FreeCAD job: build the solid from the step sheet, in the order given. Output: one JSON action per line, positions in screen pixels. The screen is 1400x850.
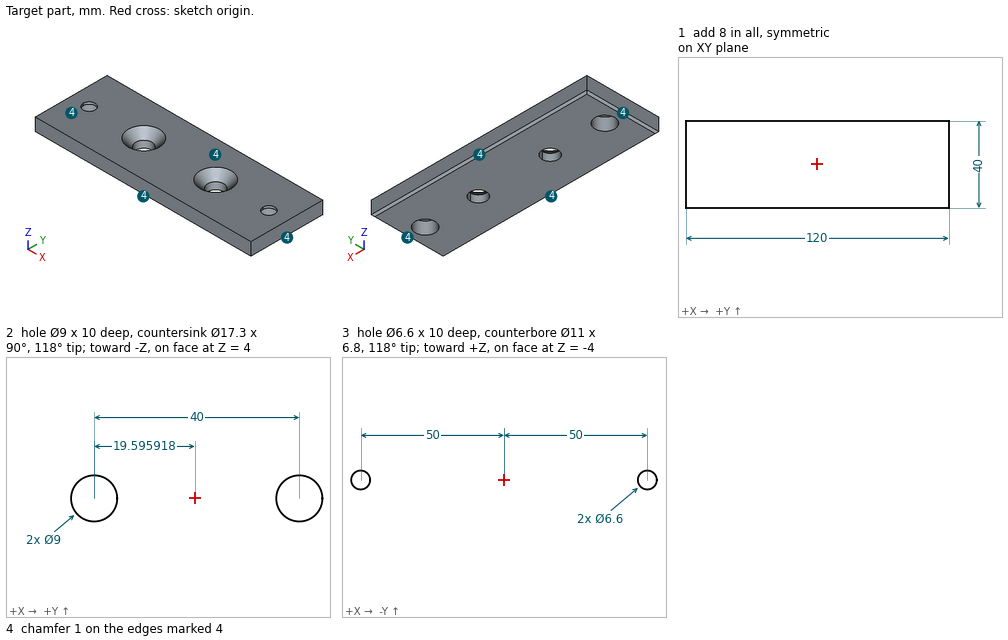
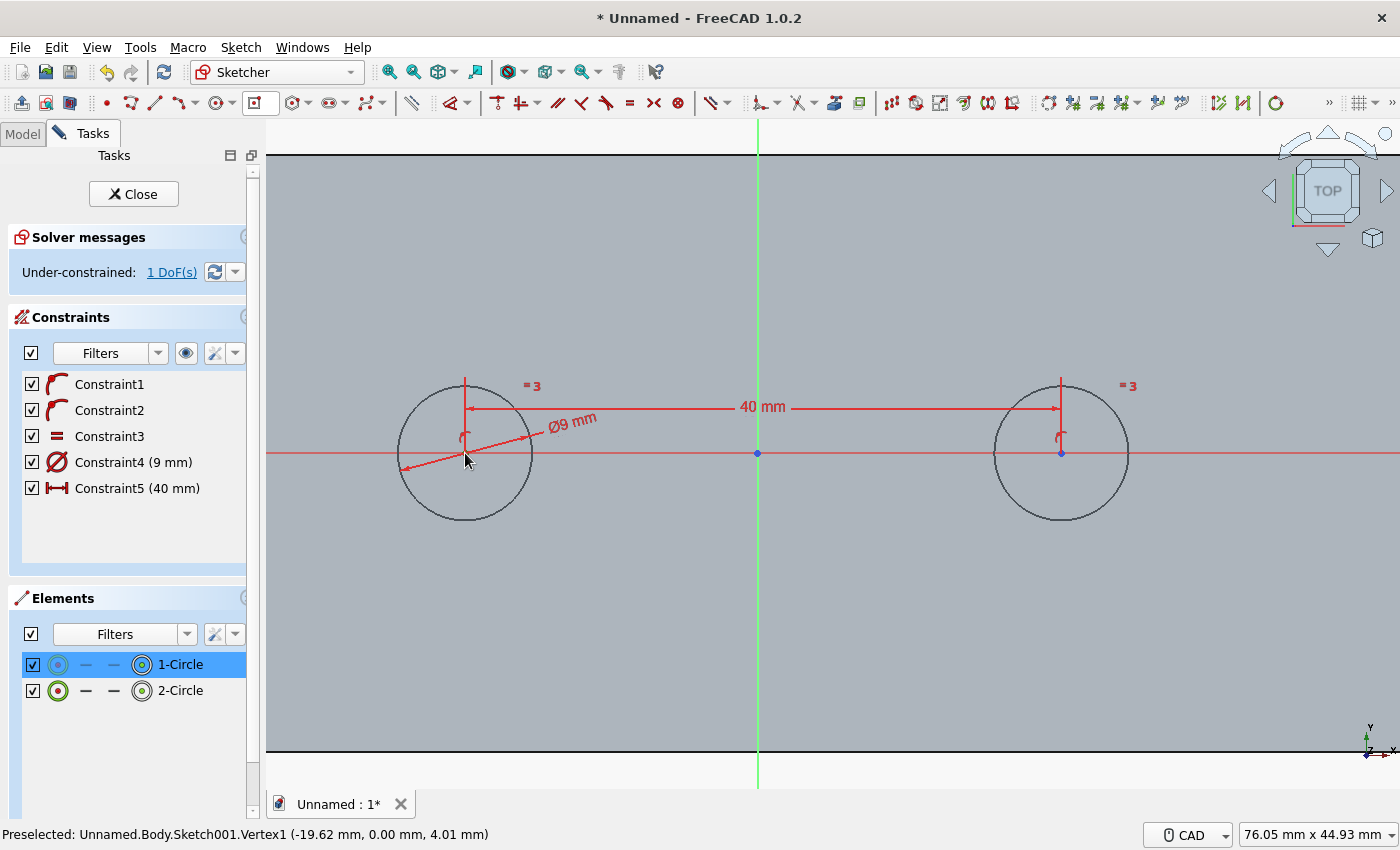
{"action": "key", "text": "l"}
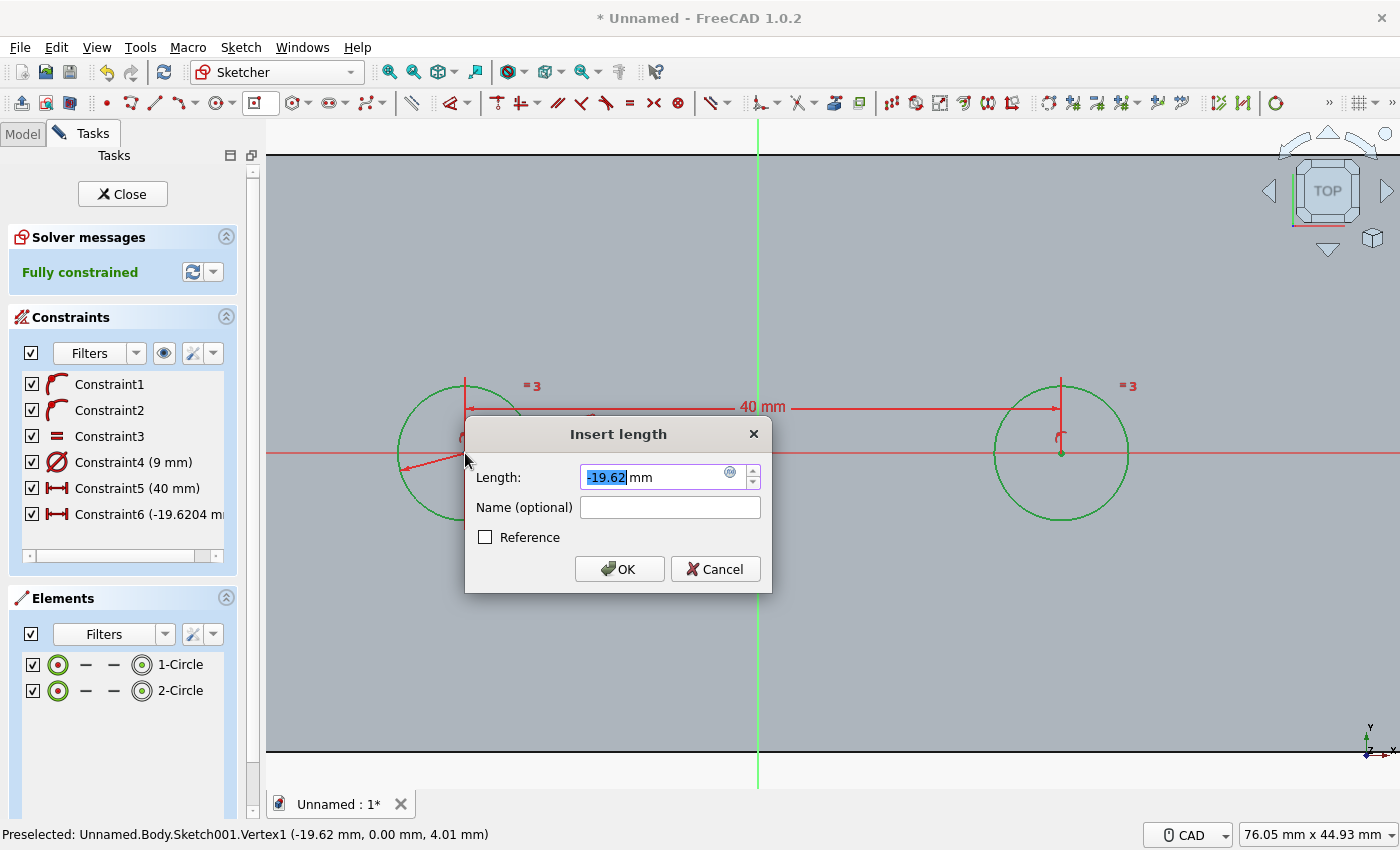
{"action": "type", "text": "-19.595918"}
{"action": "key", "text": "Return"}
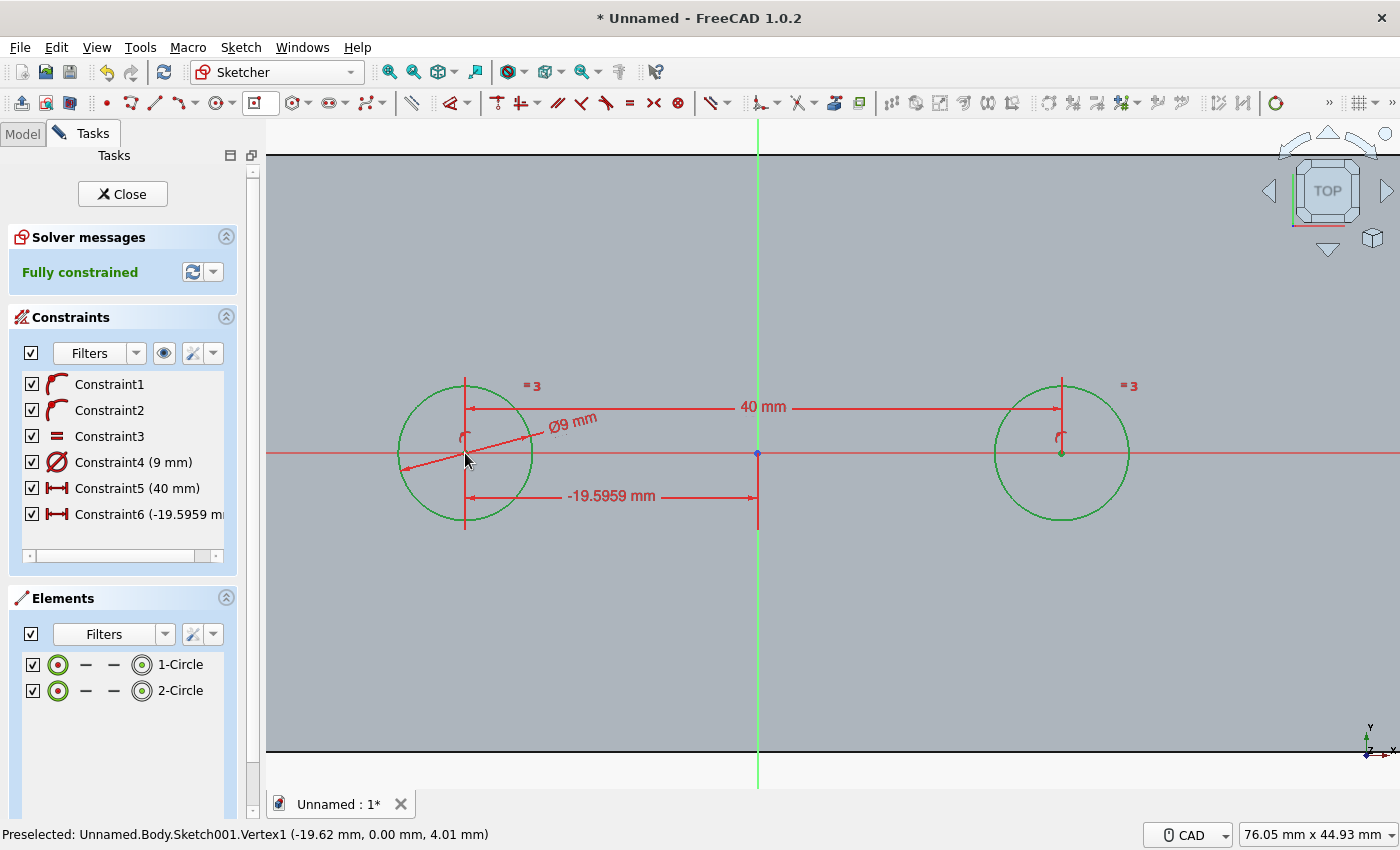
{"action": "left_click", "coordinate": [123, 194]}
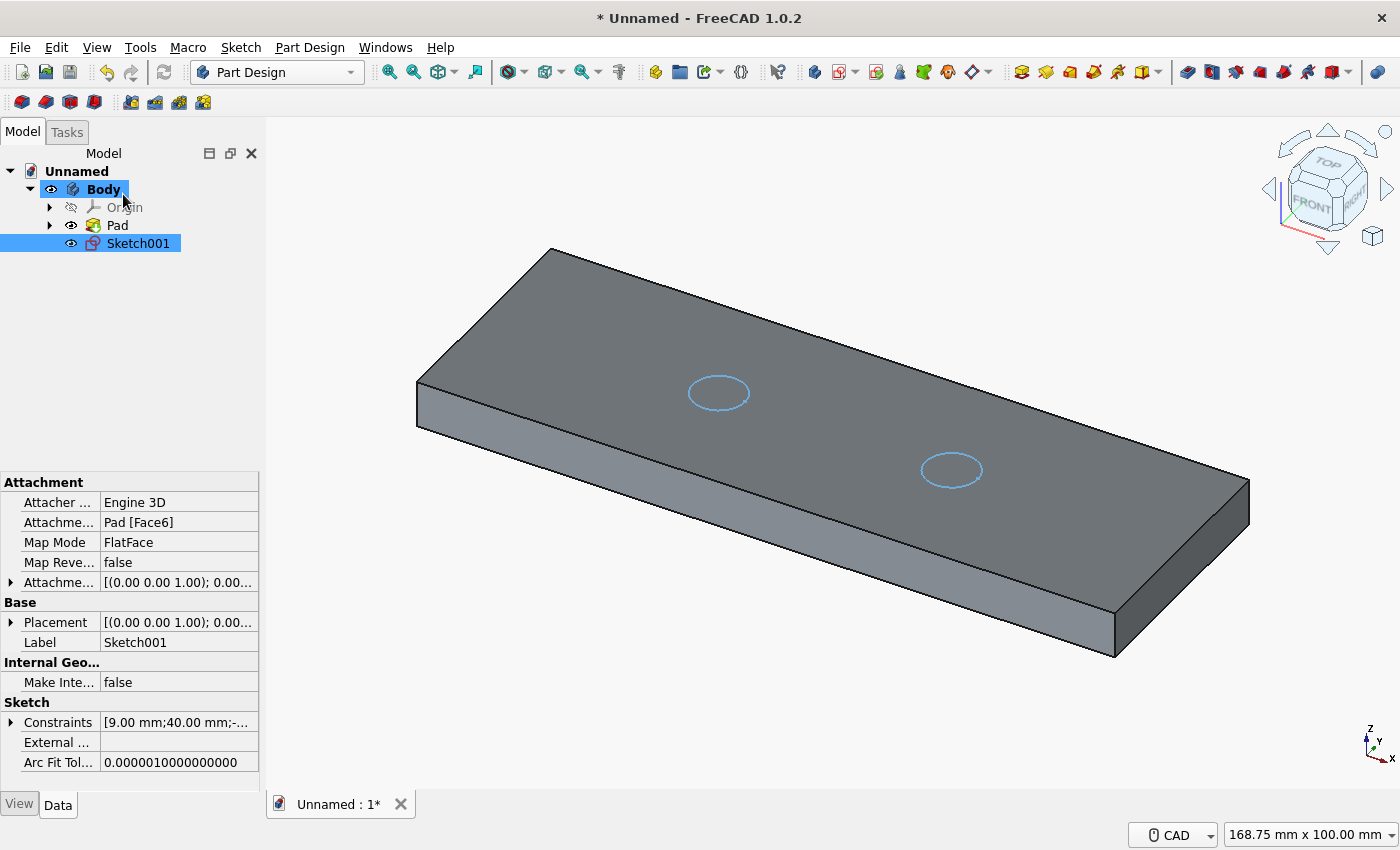
{"action": "left_click", "coordinate": [1212, 72]}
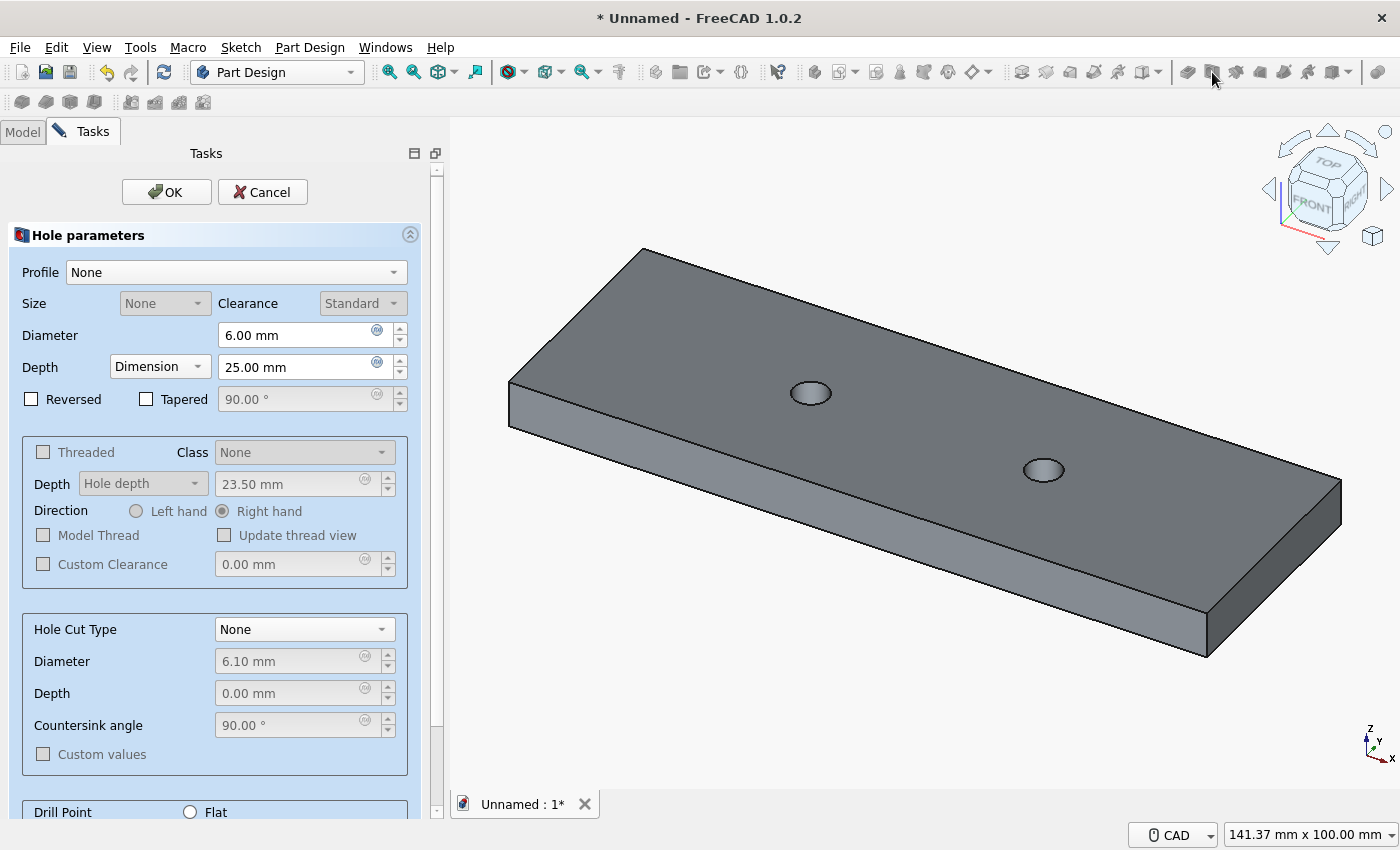
{"action": "triple_click", "coordinate": [305, 335]}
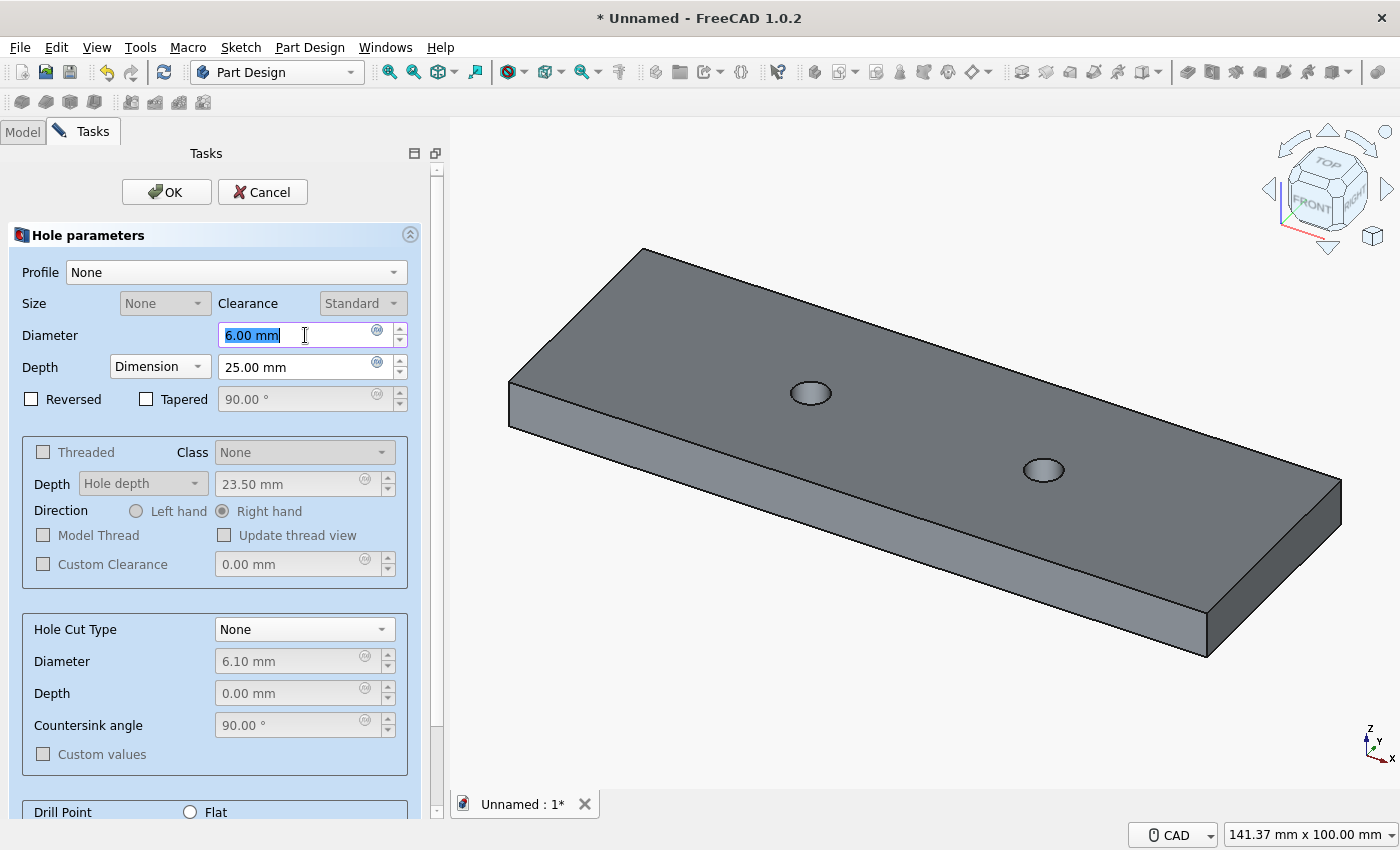
{"action": "type", "text": "9"}
{"action": "key", "text": "Tab"}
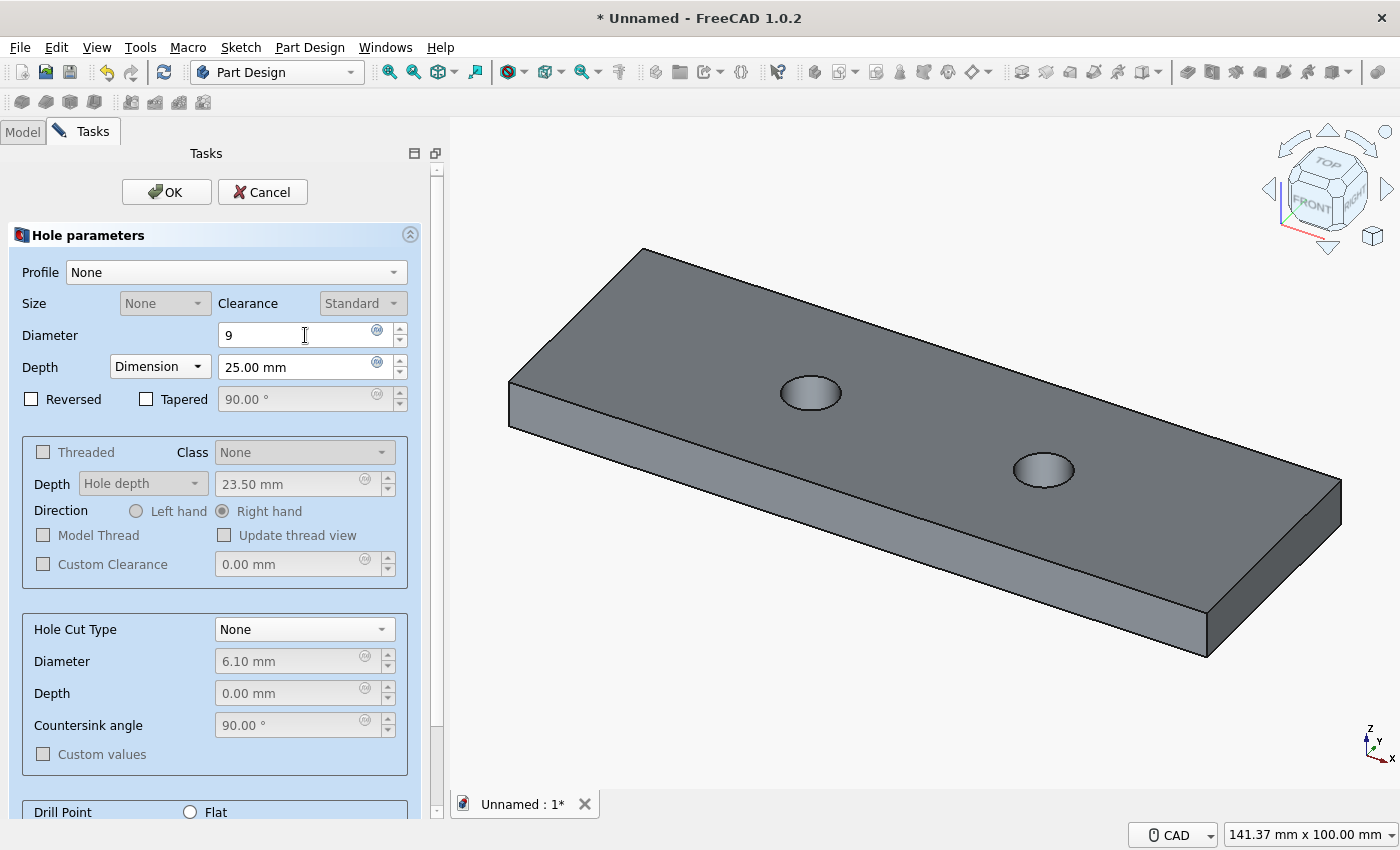
{"action": "triple_click", "coordinate": [305, 367]}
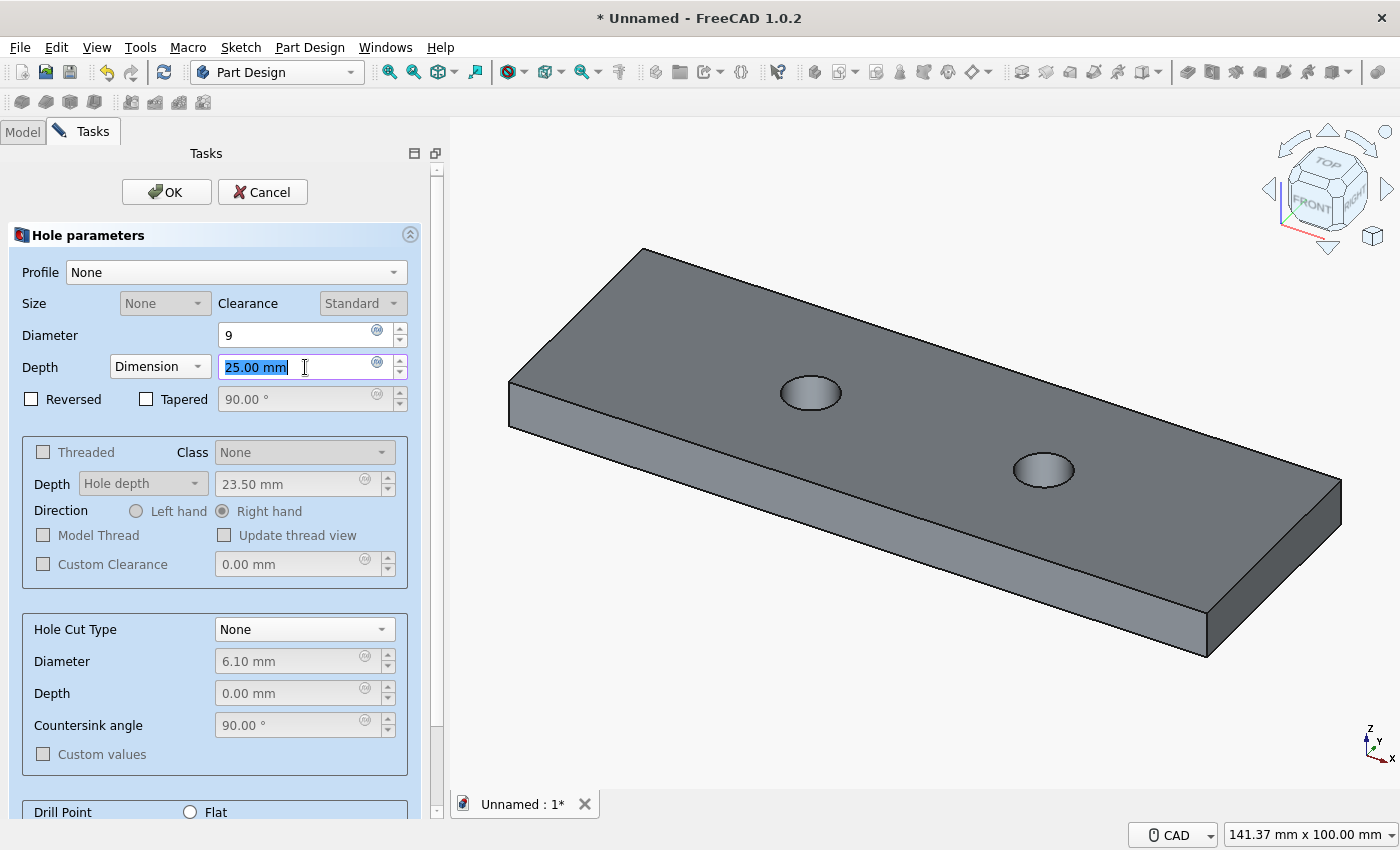
{"action": "type", "text": "10"}
{"action": "key", "text": "Tab"}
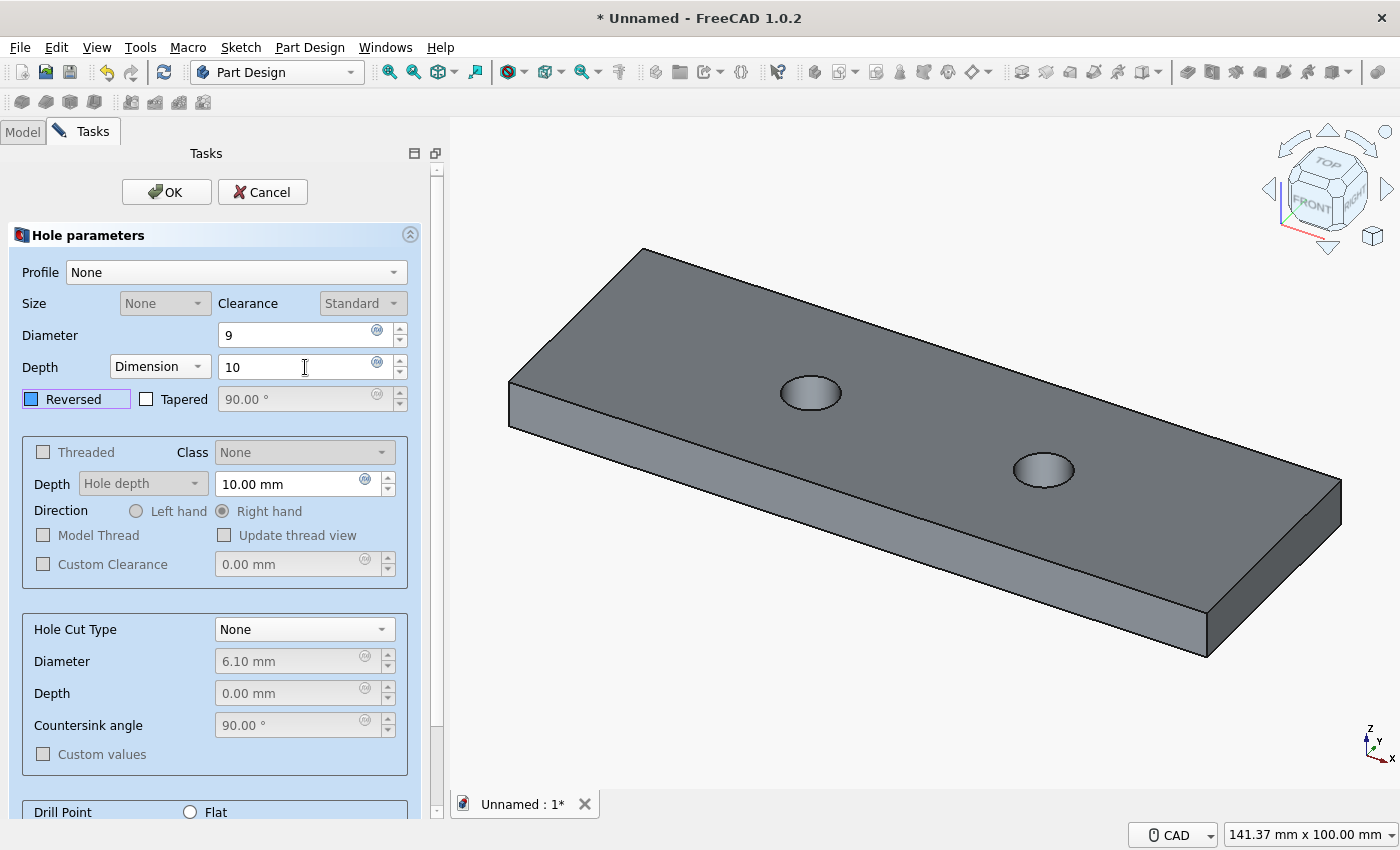
{"action": "left_click", "coordinate": [306, 630]}